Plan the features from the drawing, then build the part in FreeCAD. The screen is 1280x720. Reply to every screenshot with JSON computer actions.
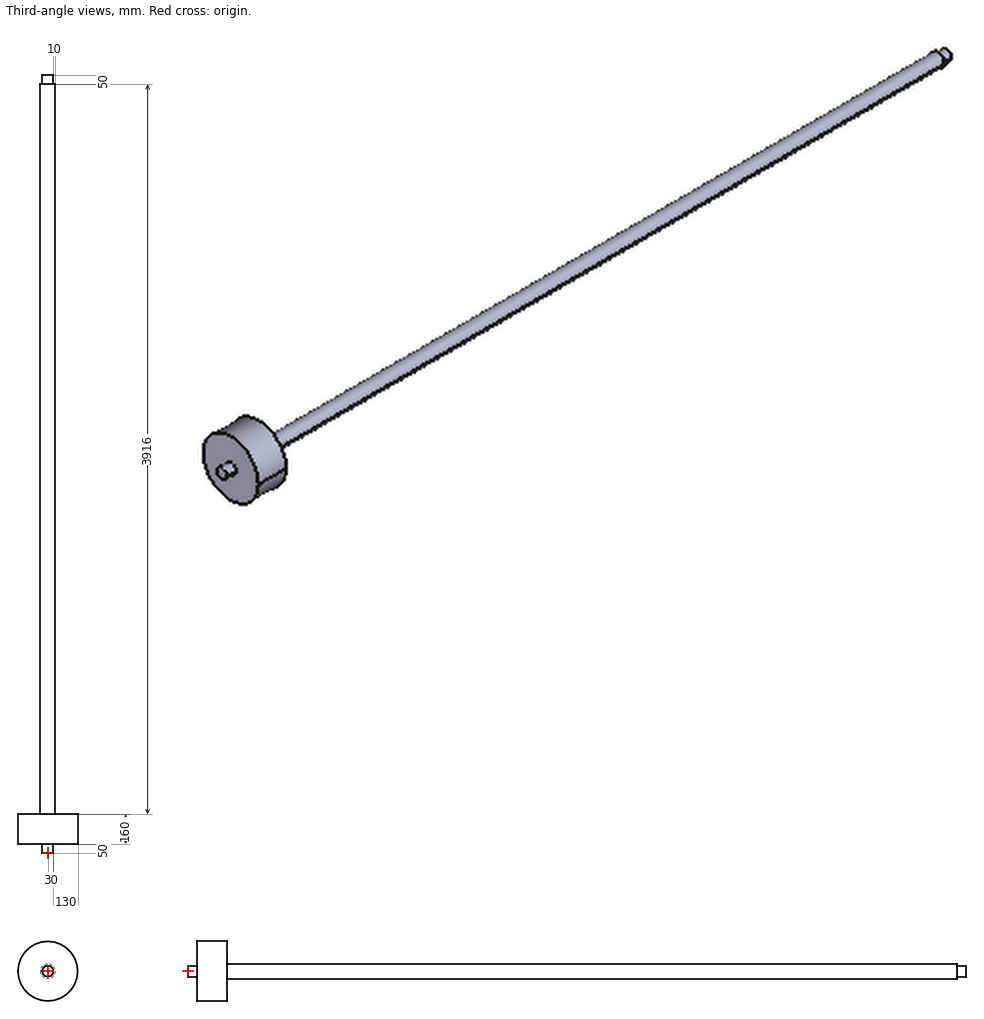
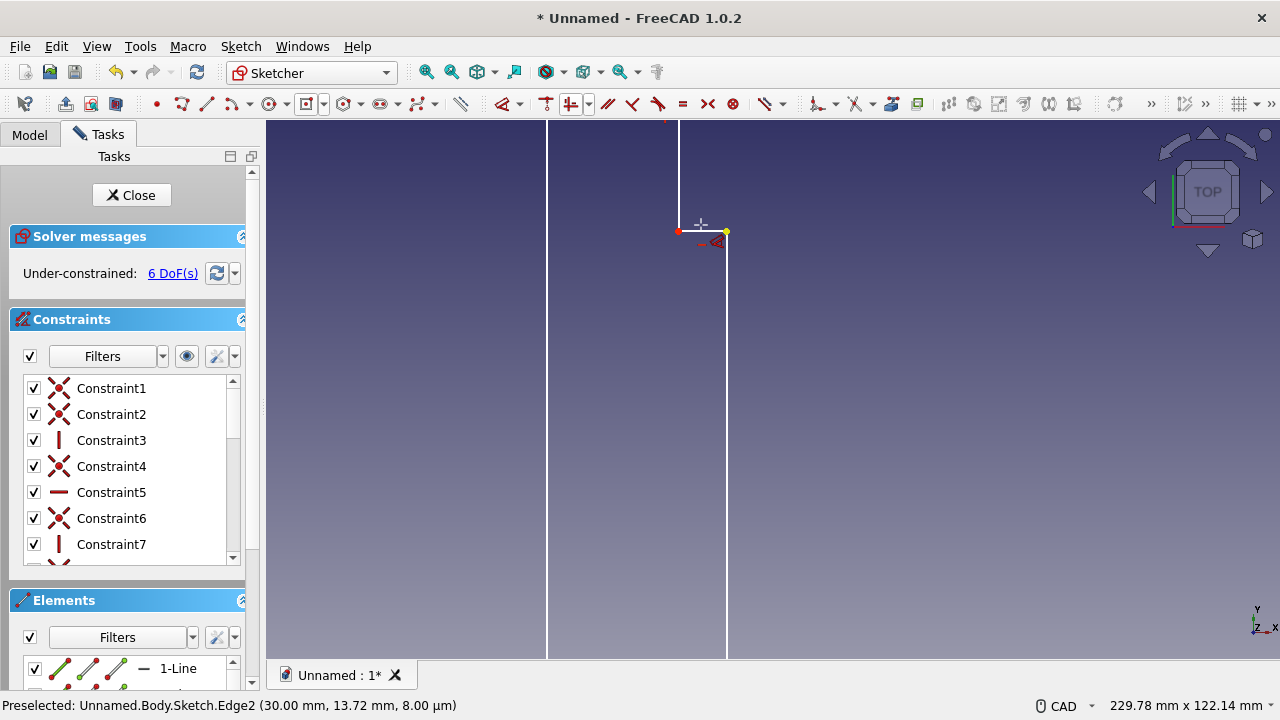
{"action": "left_click", "coordinate": [703, 231]}
{"action": "left_click", "coordinate": [703, 197]}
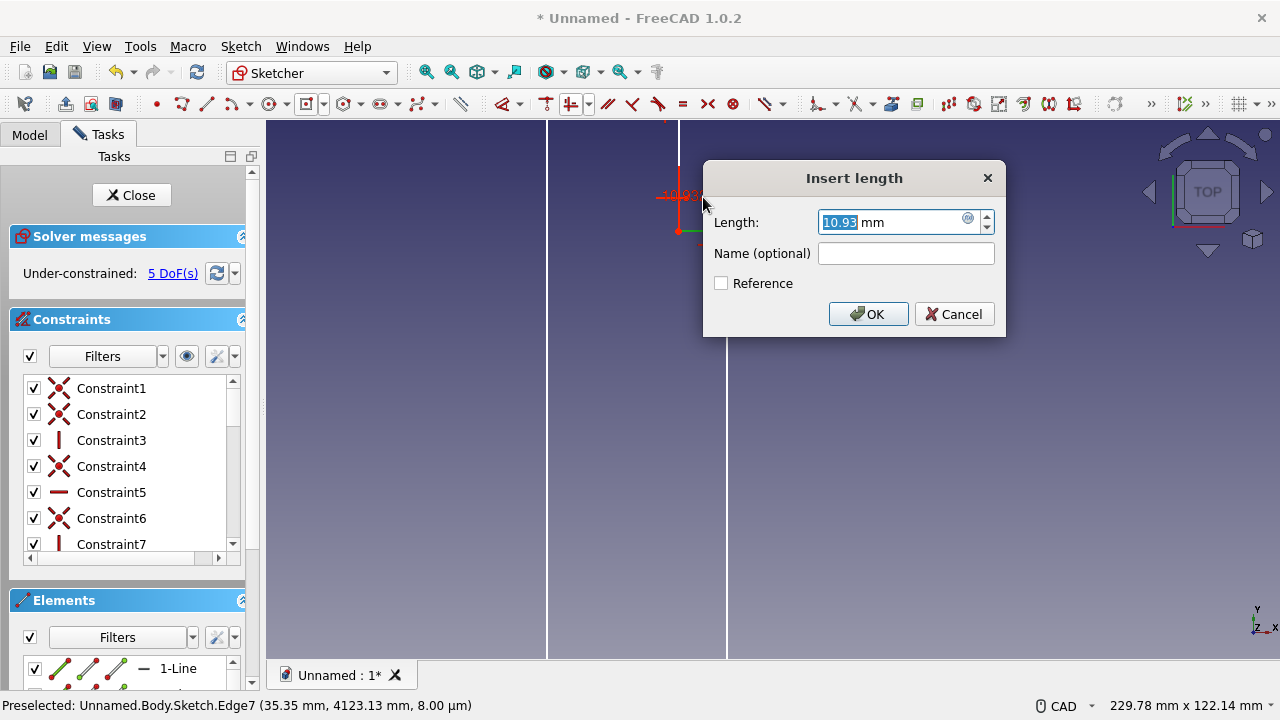
{"action": "type", "text": "10"}
{"action": "key", "text": "Return"}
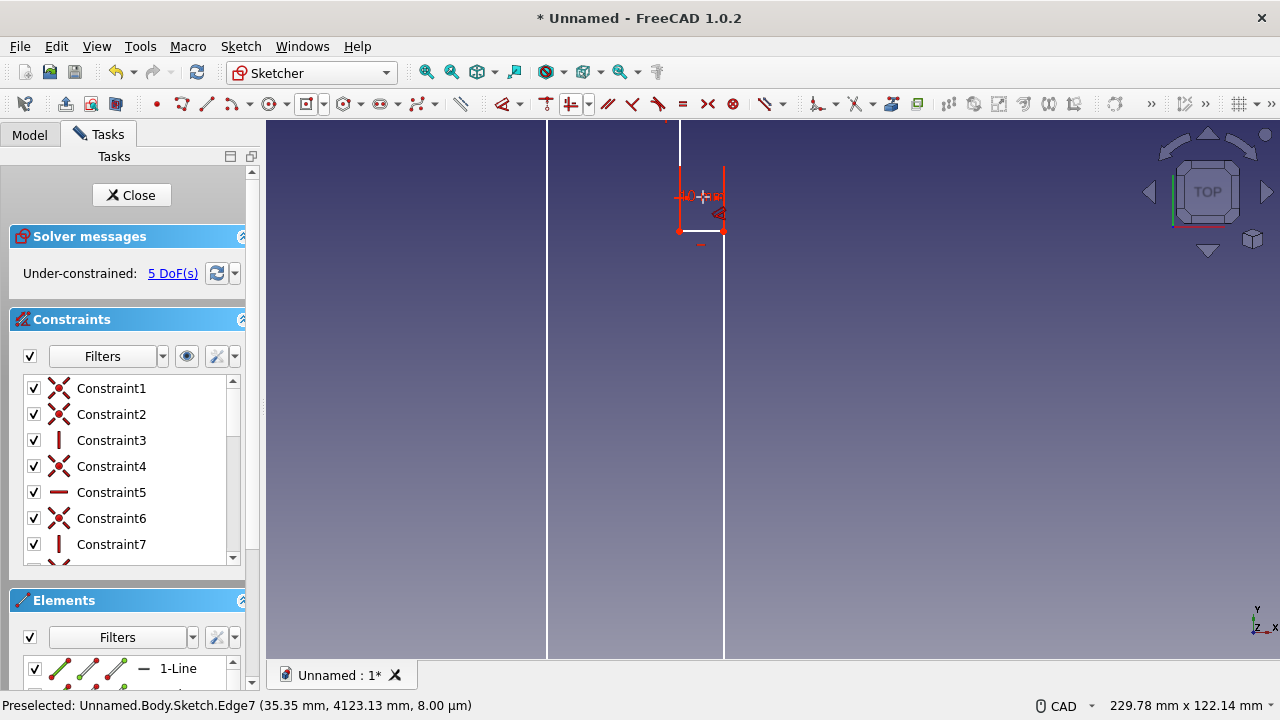
{"action": "scroll", "coordinate": [704, 390], "scroll_direction": "down", "scroll_amount": 15}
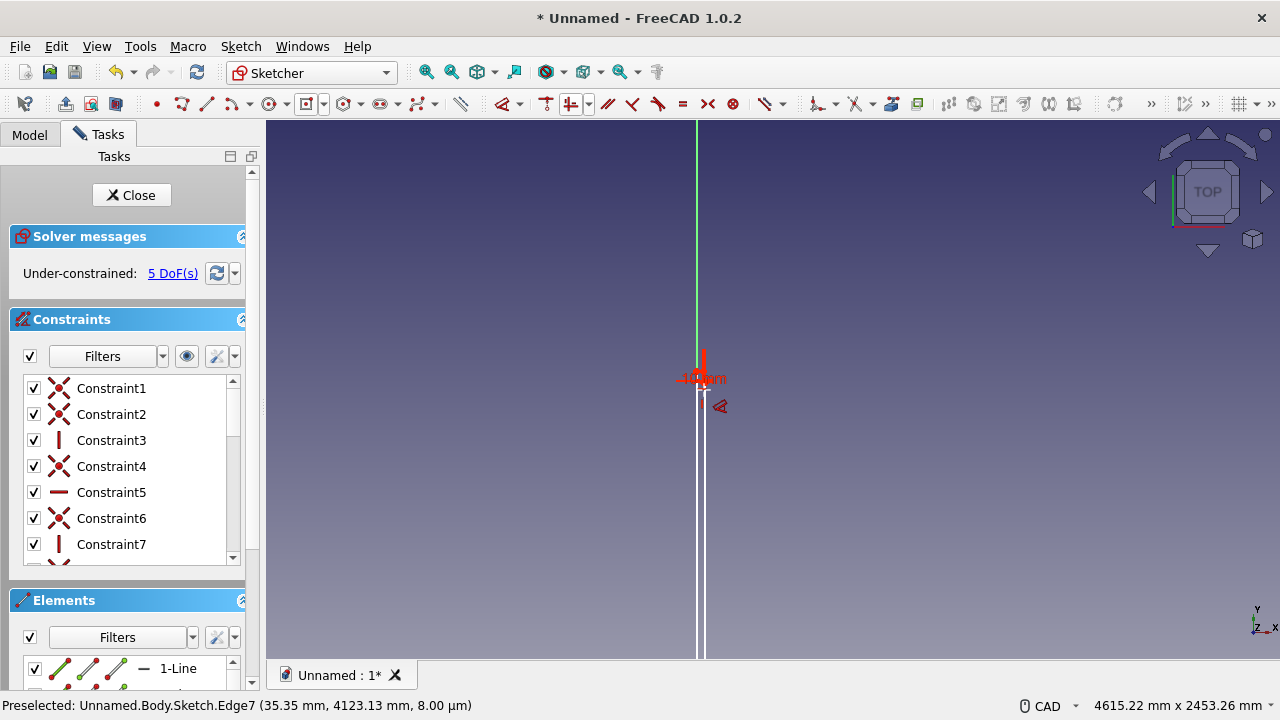
{"action": "scroll", "coordinate": [699, 148], "scroll_direction": "down", "scroll_amount": 5}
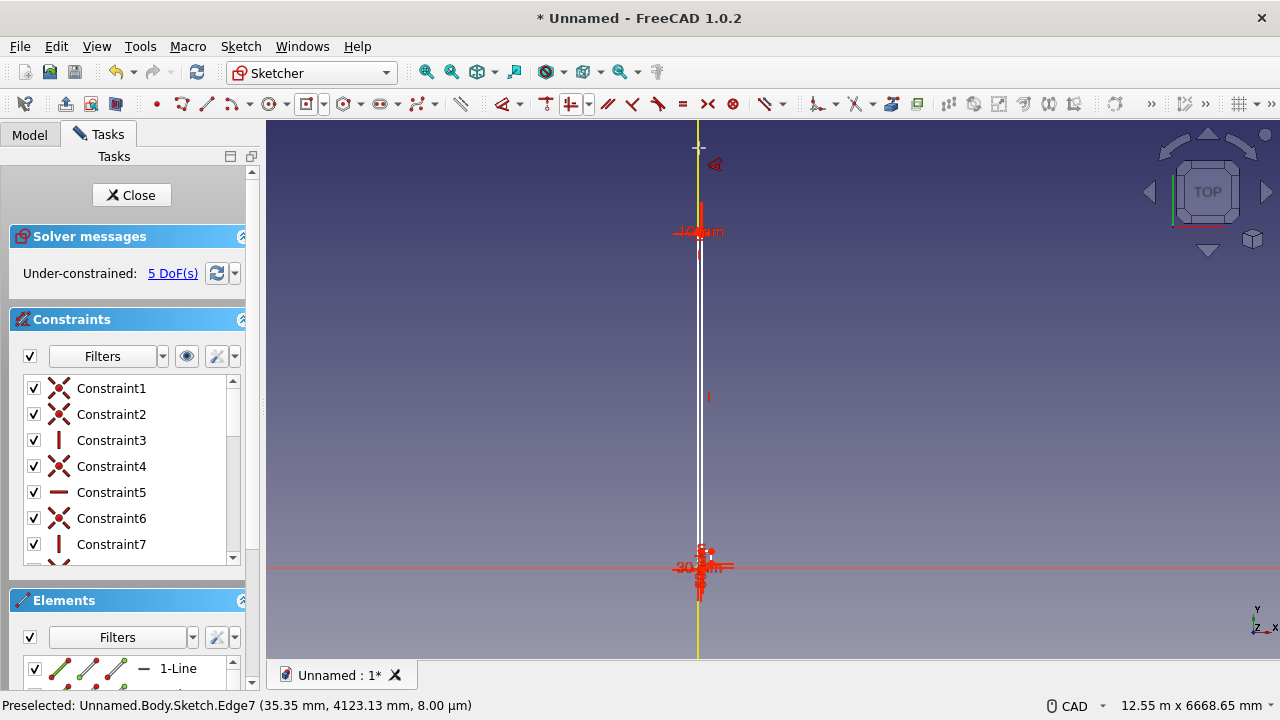
{"action": "scroll", "coordinate": [701, 233], "scroll_direction": "up", "scroll_amount": 13}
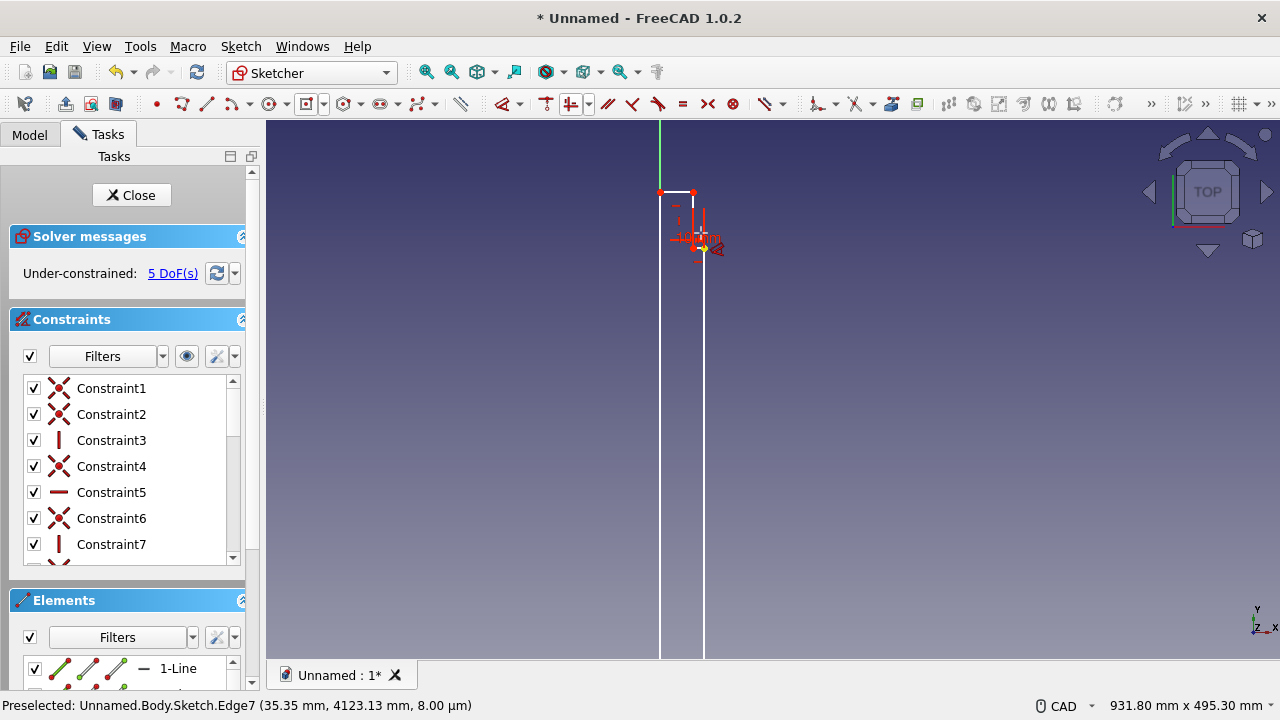
{"action": "left_click", "coordinate": [693, 232]}
{"action": "left_click", "coordinate": [727, 208]}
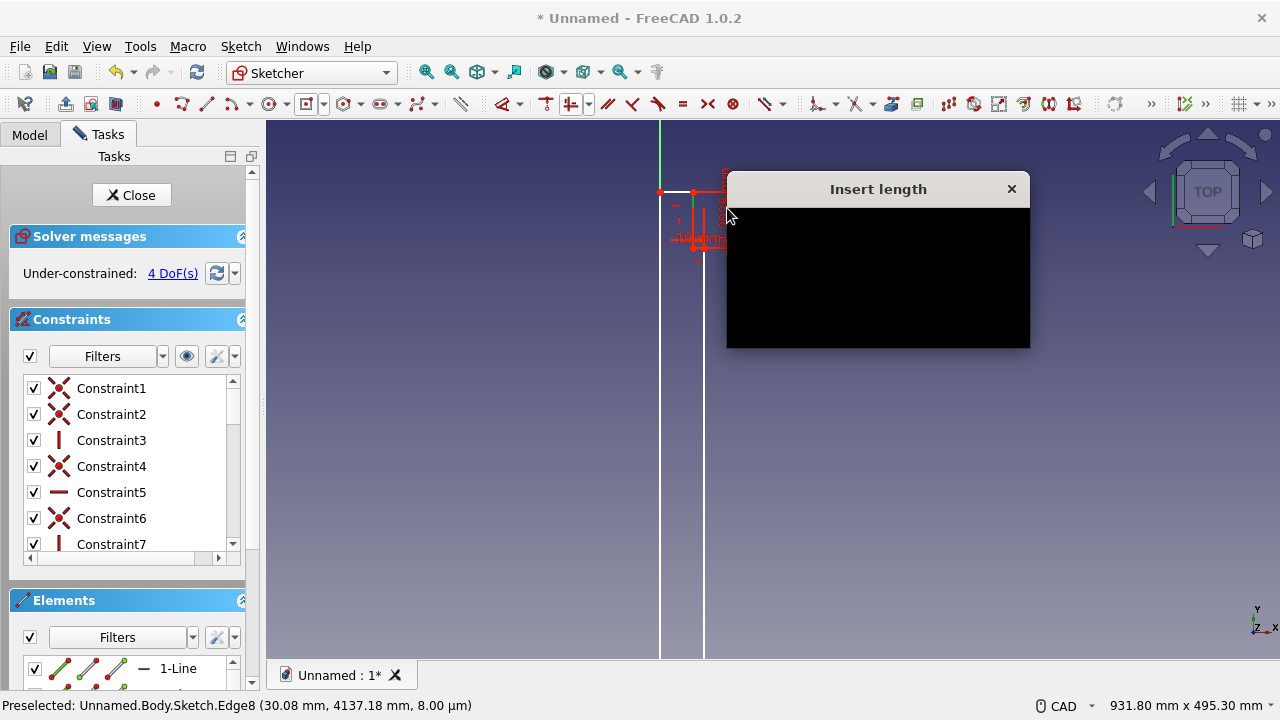
{"action": "type", "text": "50"}
{"action": "key", "text": "Return"}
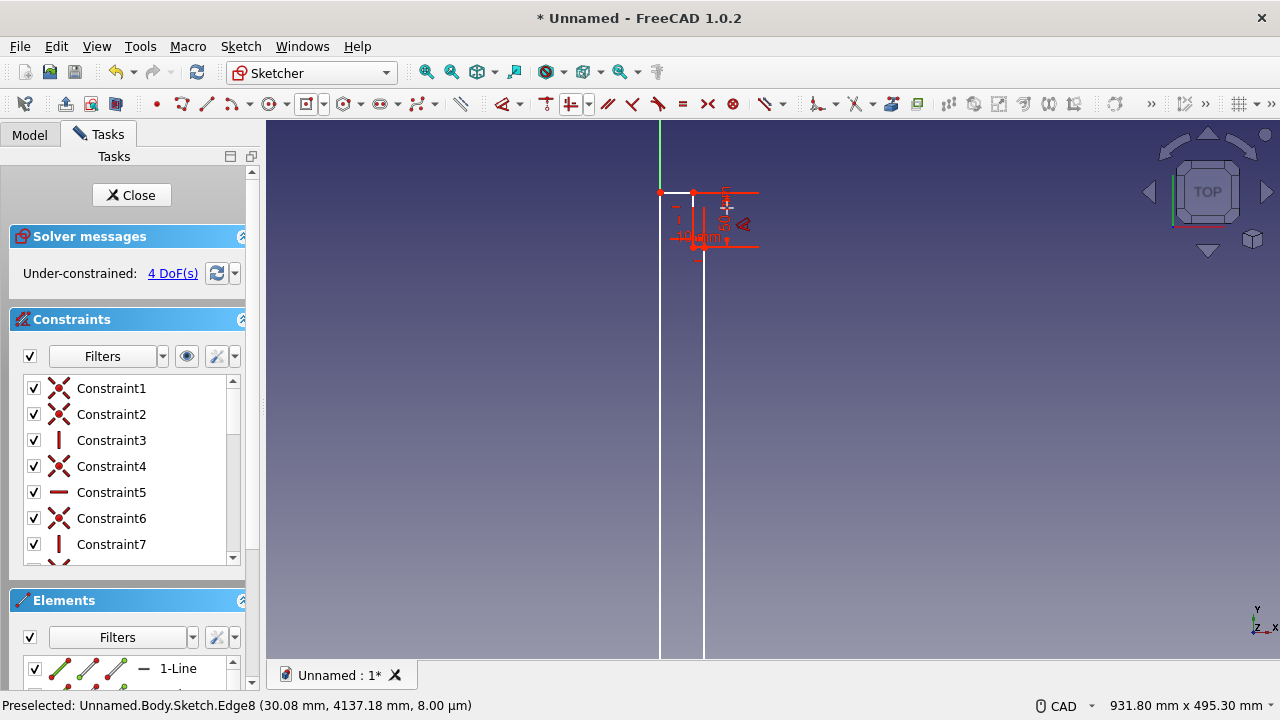
{"action": "left_click", "coordinate": [683, 193]}
{"action": "left_click", "coordinate": [677, 159]}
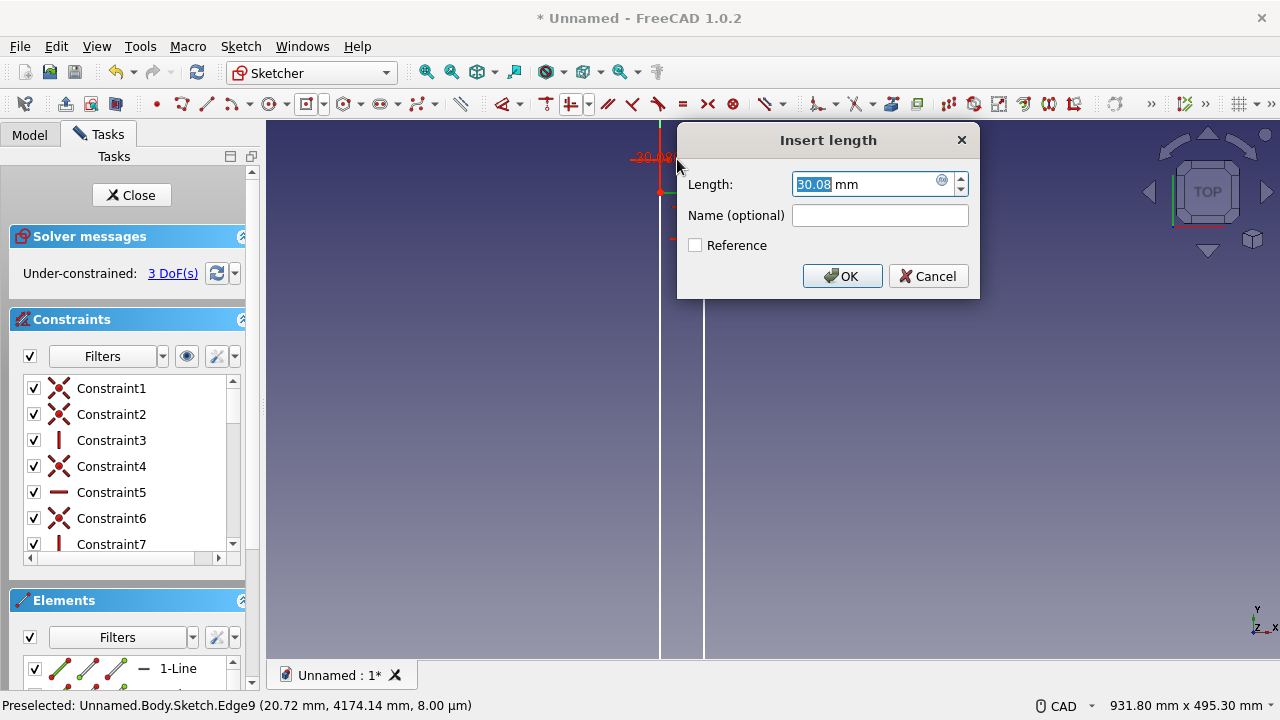
{"action": "type", "text": "30"}
{"action": "key", "text": "Return"}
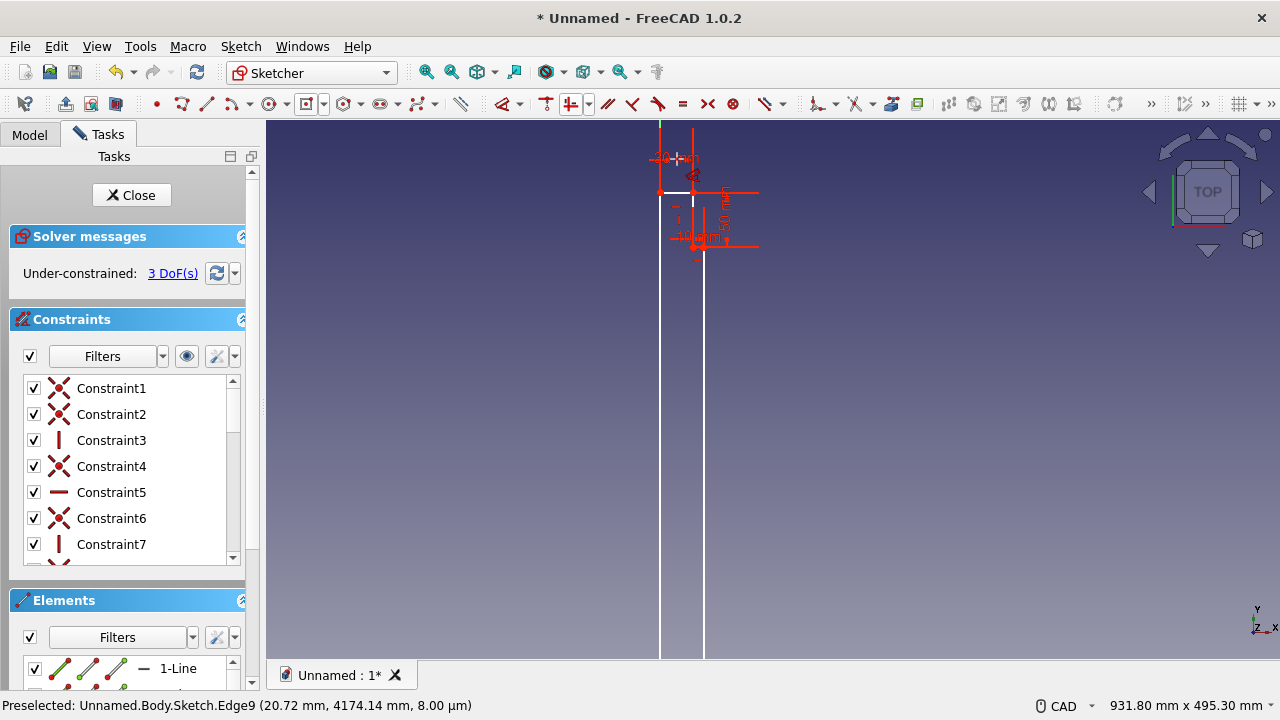
{"action": "scroll", "coordinate": [701, 223], "scroll_direction": "down", "scroll_amount": 13}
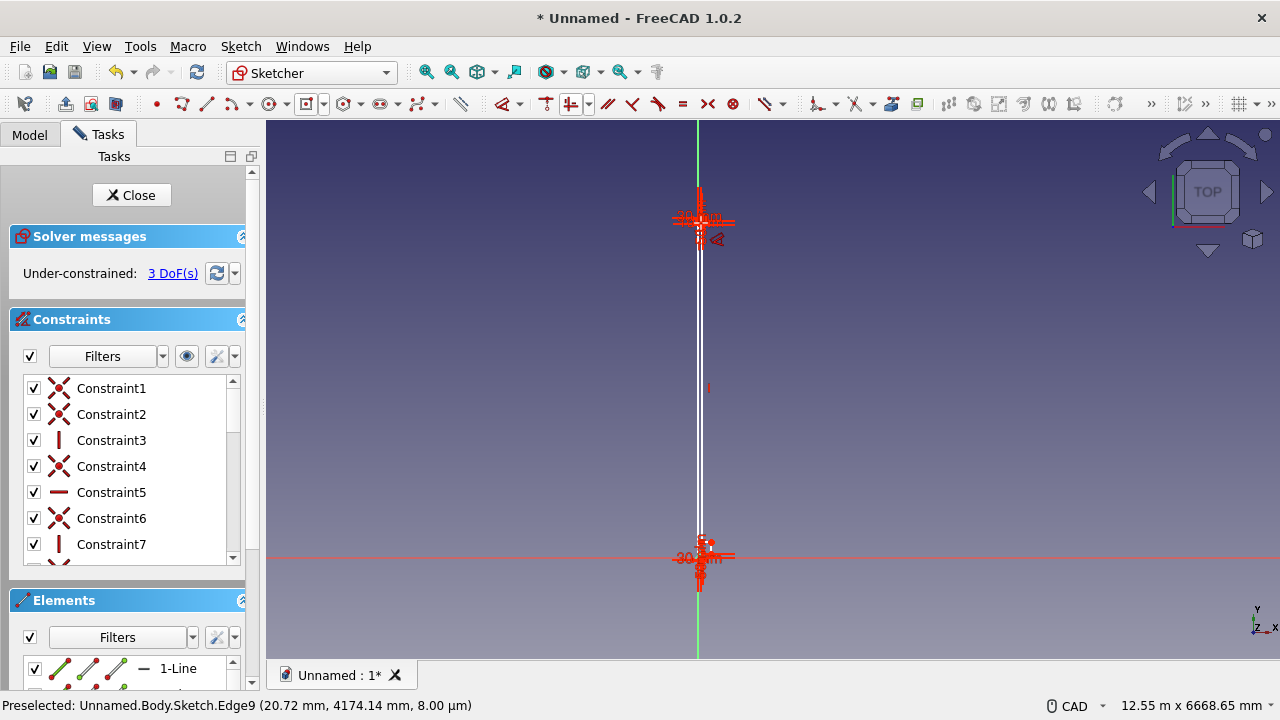
{"action": "scroll", "coordinate": [704, 554], "scroll_direction": "up", "scroll_amount": 8}